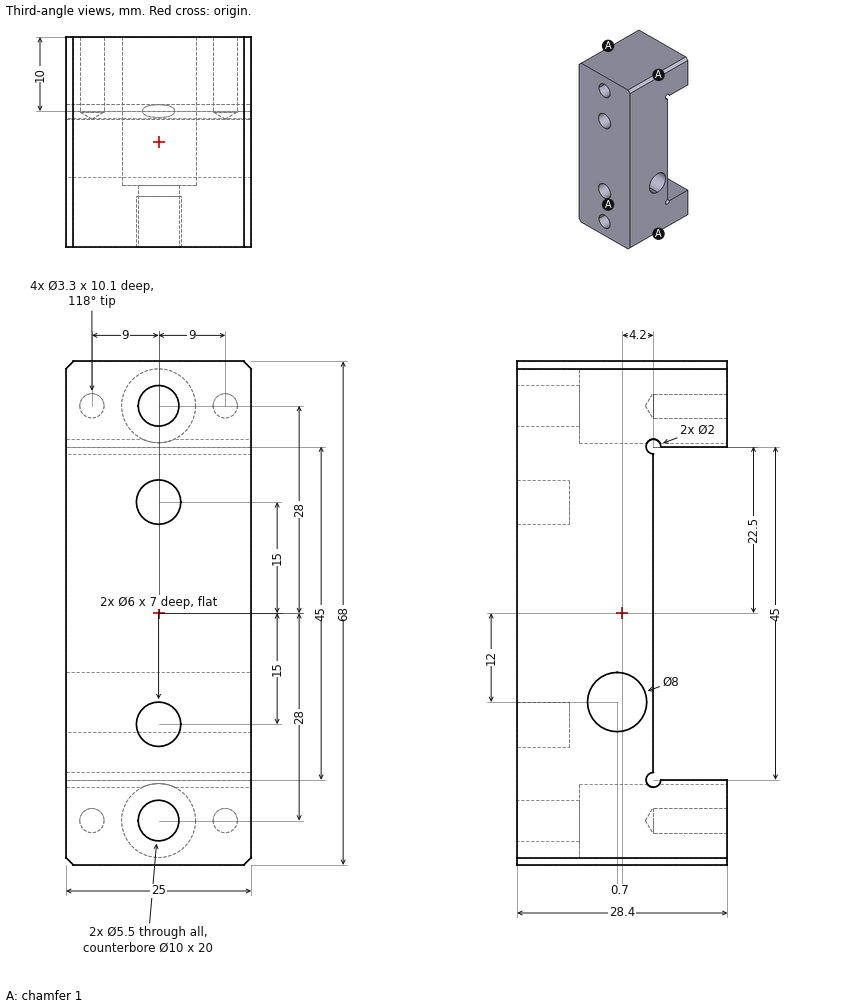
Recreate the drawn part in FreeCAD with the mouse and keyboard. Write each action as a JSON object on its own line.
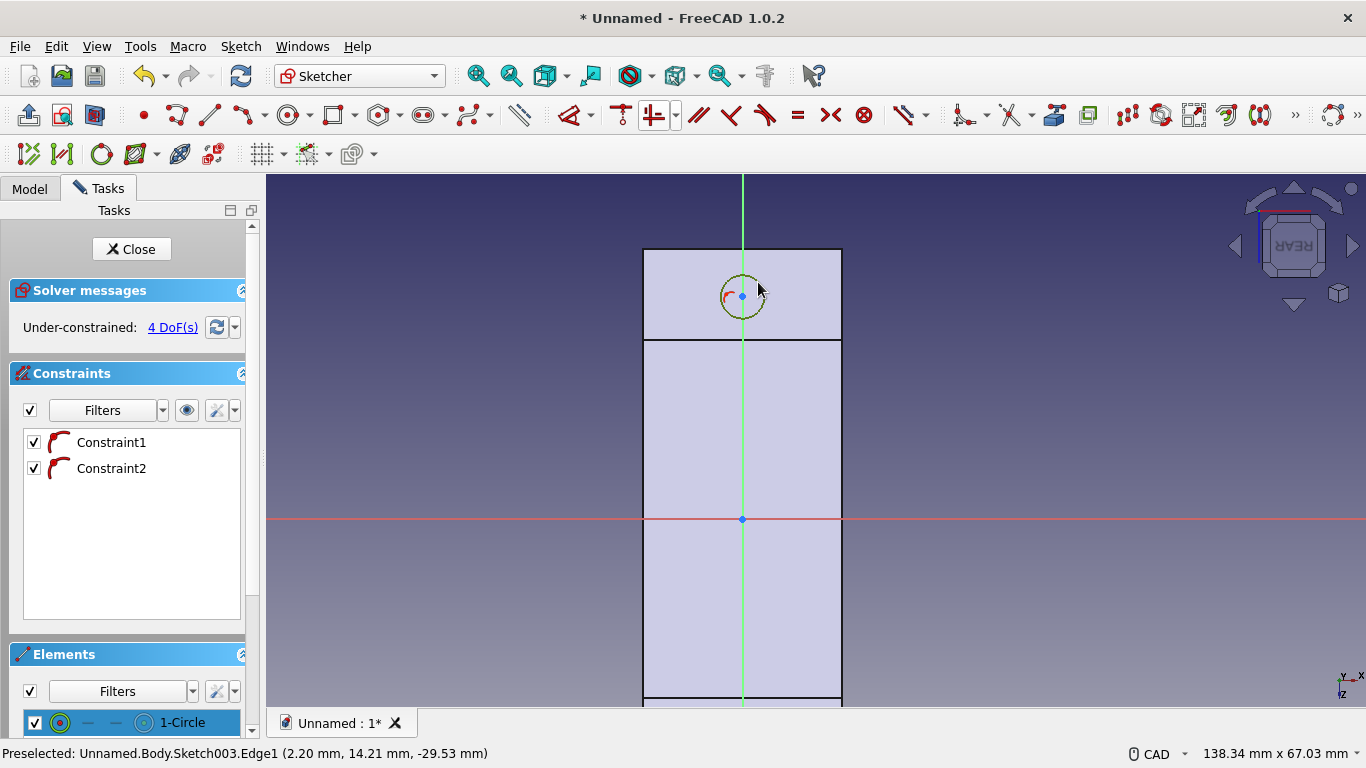
{"action": "scroll", "coordinate": [758, 281], "scroll_direction": "down", "scroll_amount": 2}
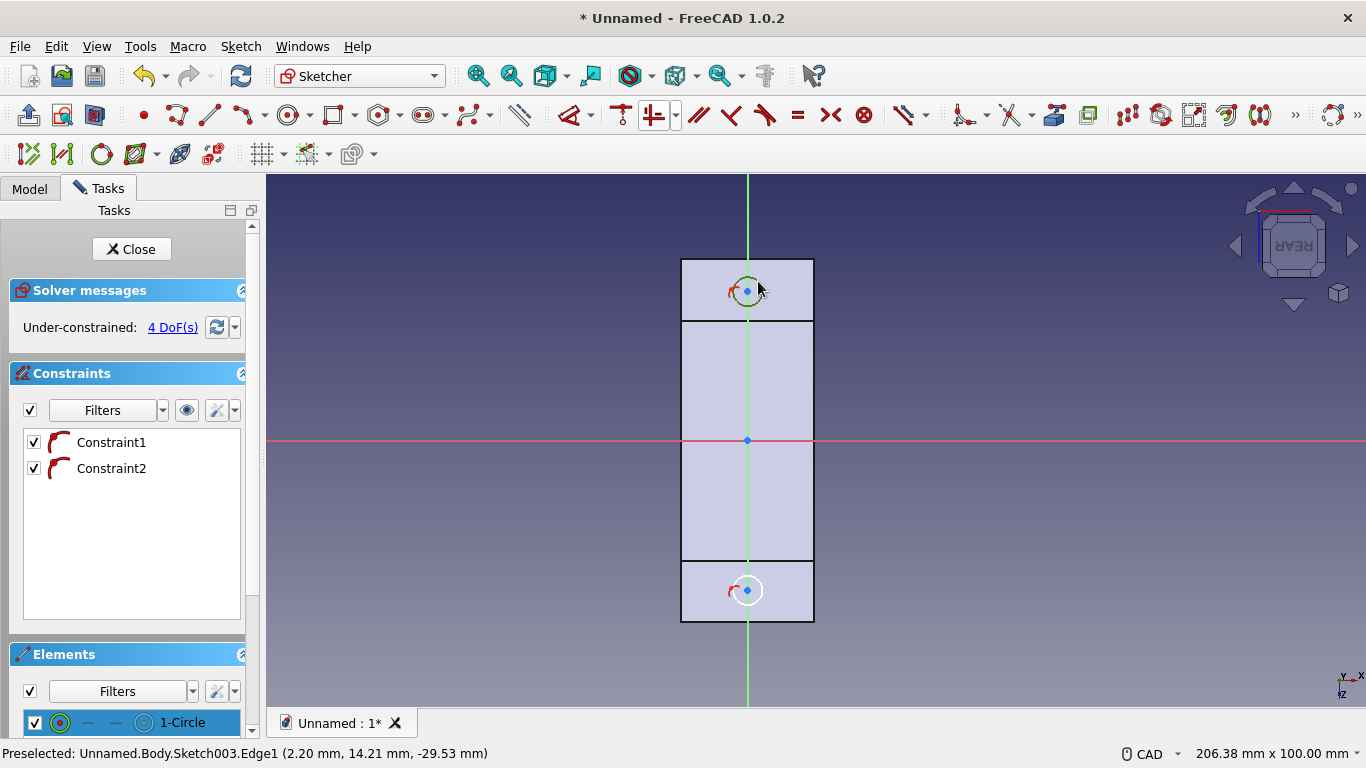
{"action": "scroll", "coordinate": [758, 580], "scroll_direction": "up", "scroll_amount": 2}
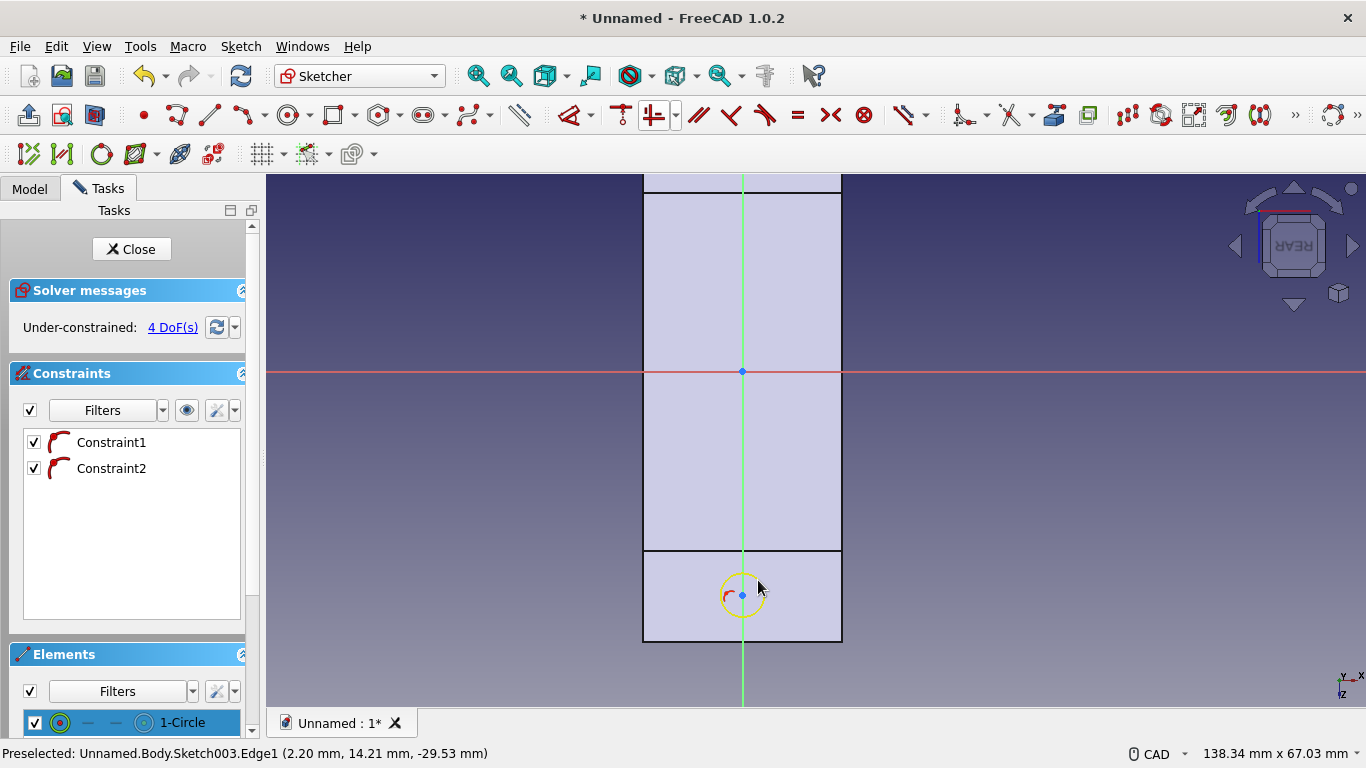
{"action": "left_click", "coordinate": [758, 580]}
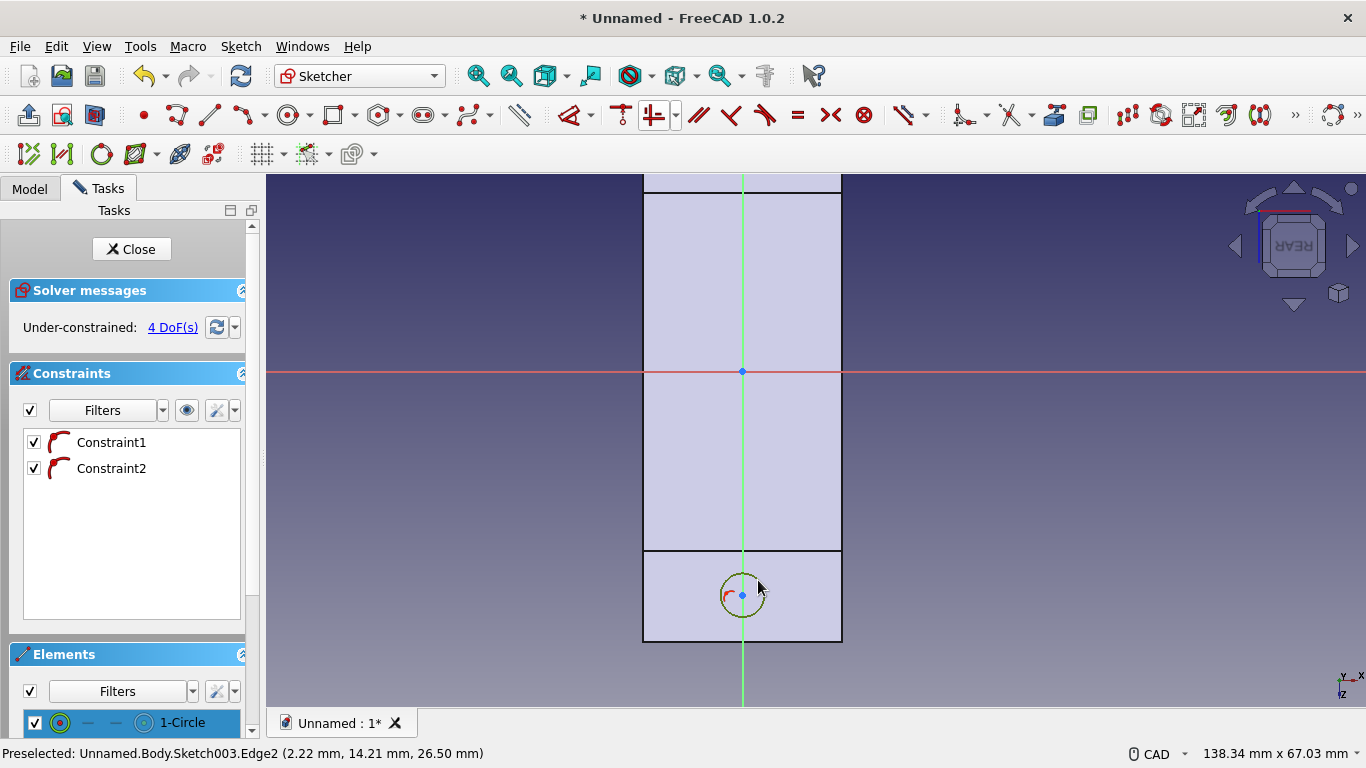
{"action": "key", "text": "e"}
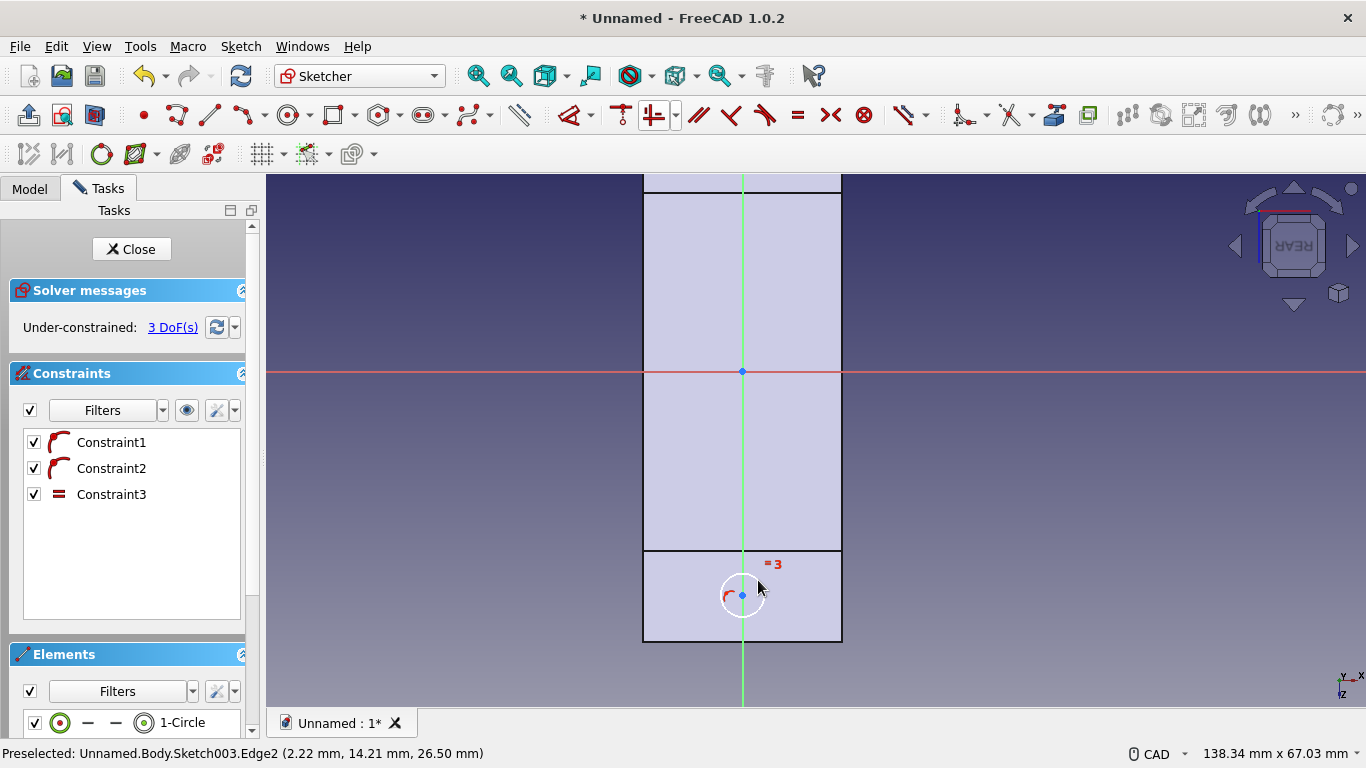
{"action": "key", "text": "d"}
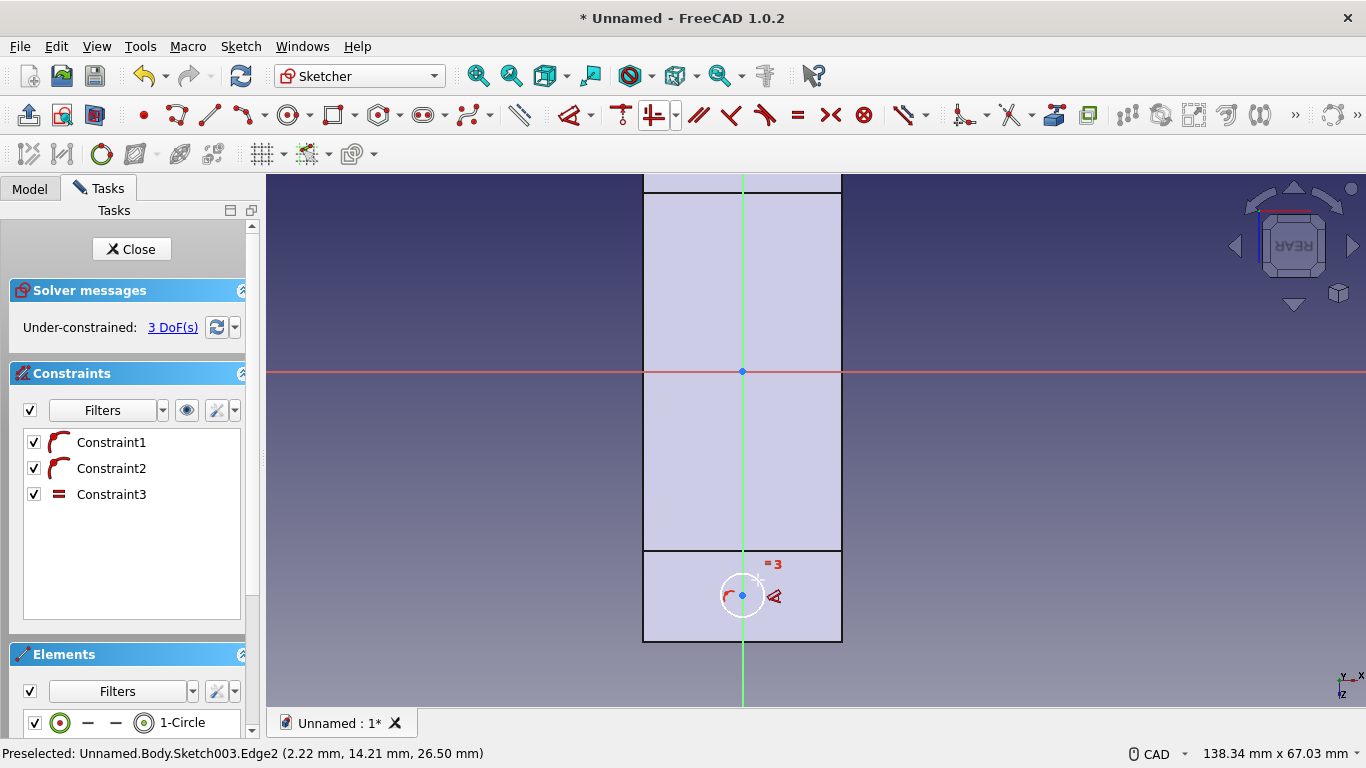
{"action": "scroll", "coordinate": [758, 580], "scroll_direction": "down", "scroll_amount": 2}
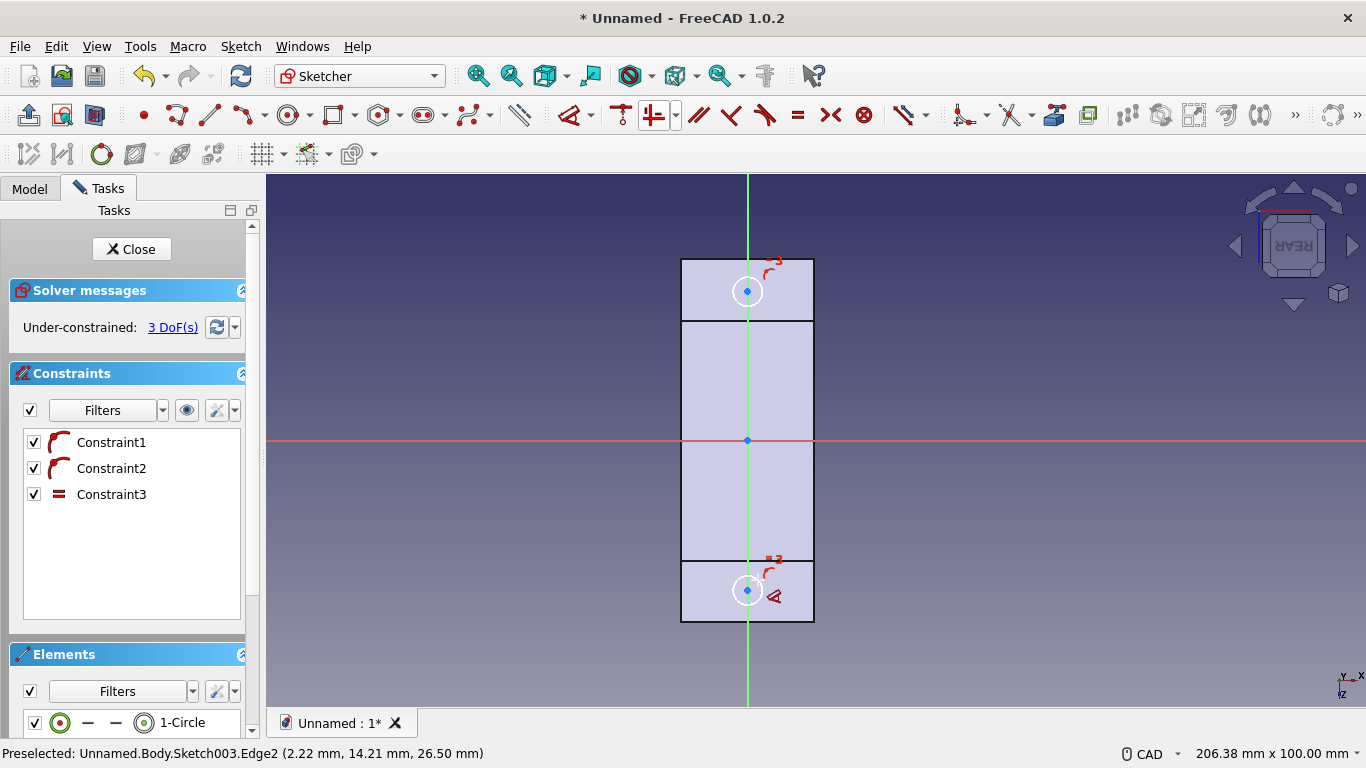
{"action": "scroll", "coordinate": [758, 281], "scroll_direction": "up", "scroll_amount": 2}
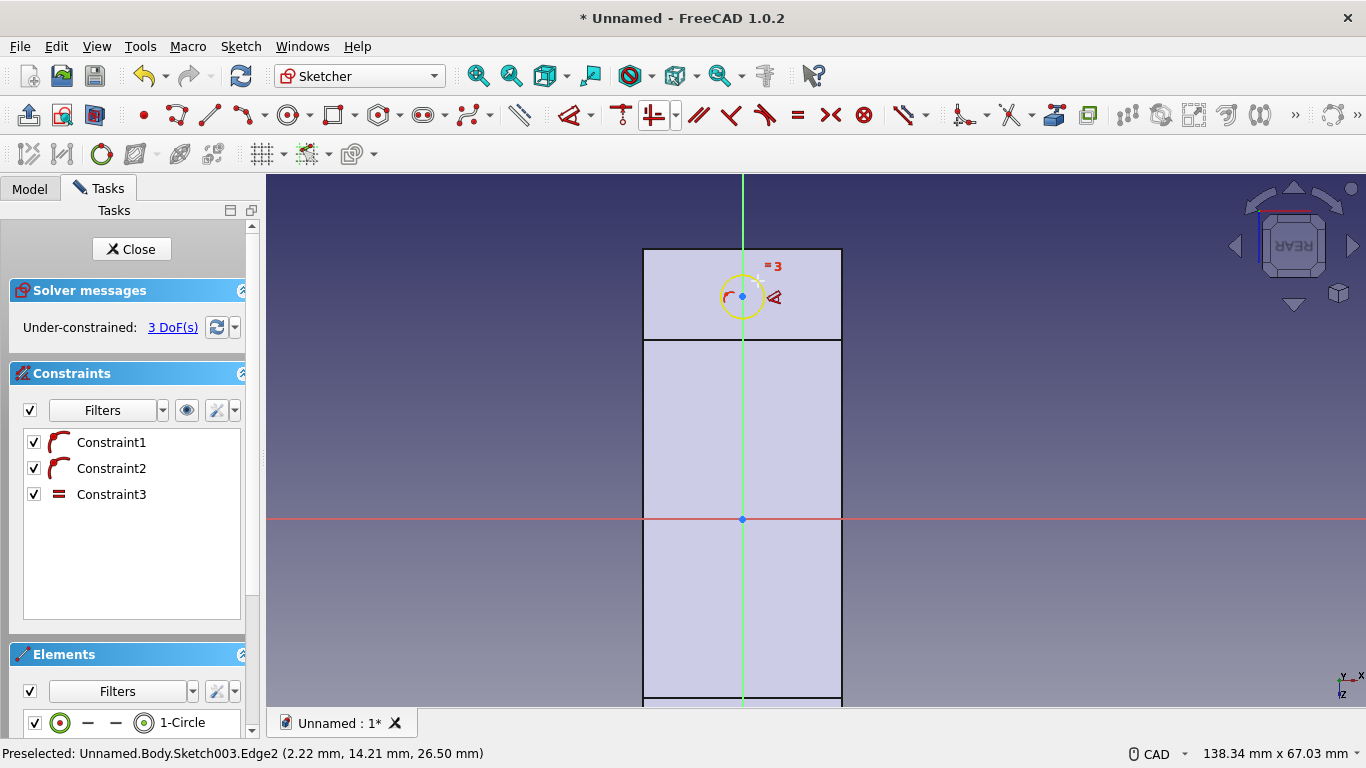
{"action": "left_click", "coordinate": [758, 282]}
{"action": "left_click", "coordinate": [781, 260]}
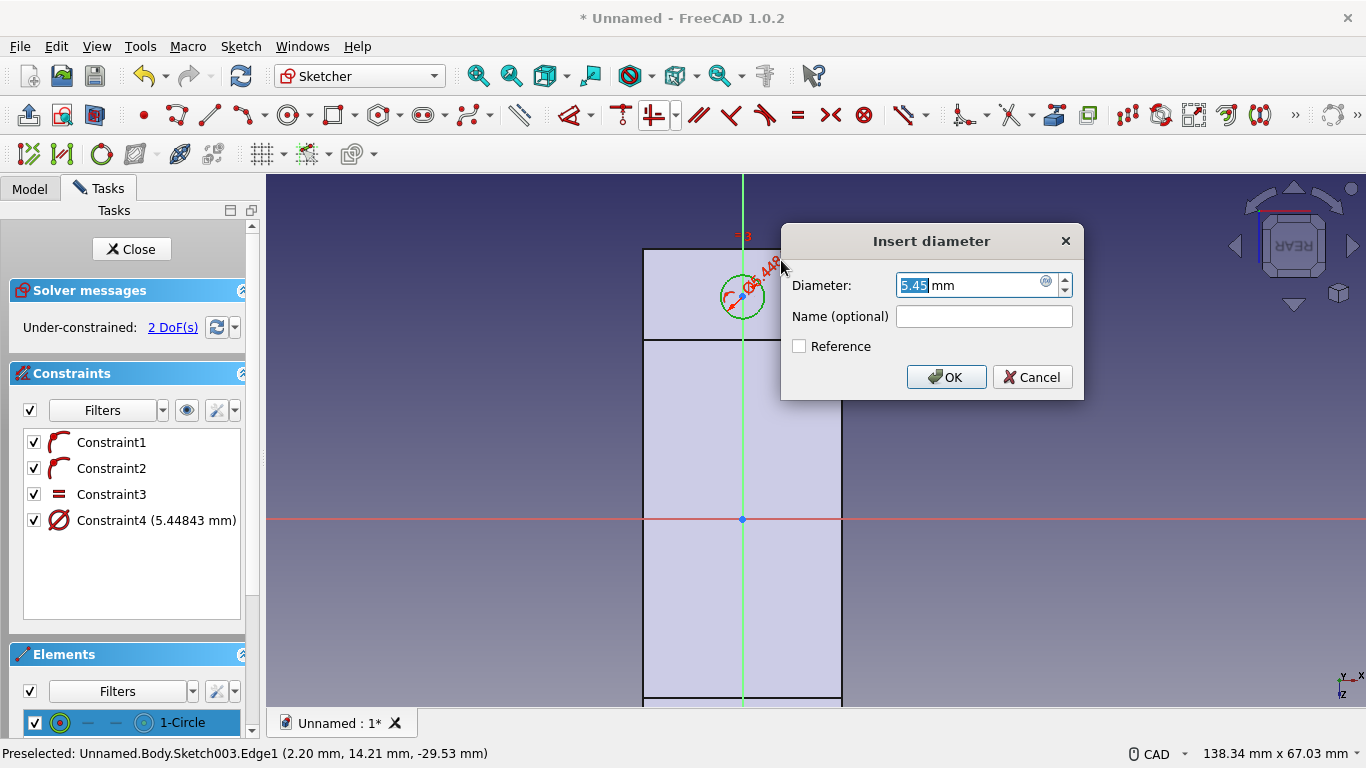
{"action": "type", "text": "5.5"}
{"action": "key", "text": "Return"}